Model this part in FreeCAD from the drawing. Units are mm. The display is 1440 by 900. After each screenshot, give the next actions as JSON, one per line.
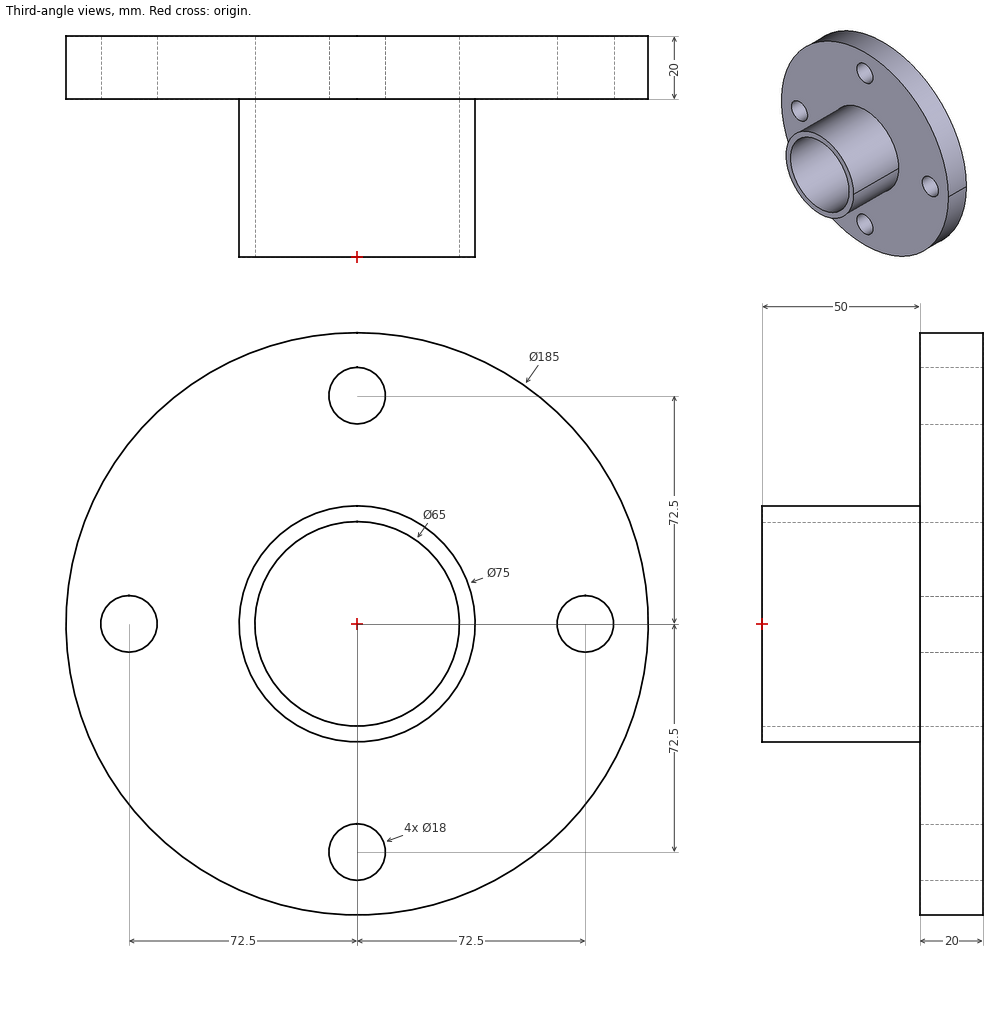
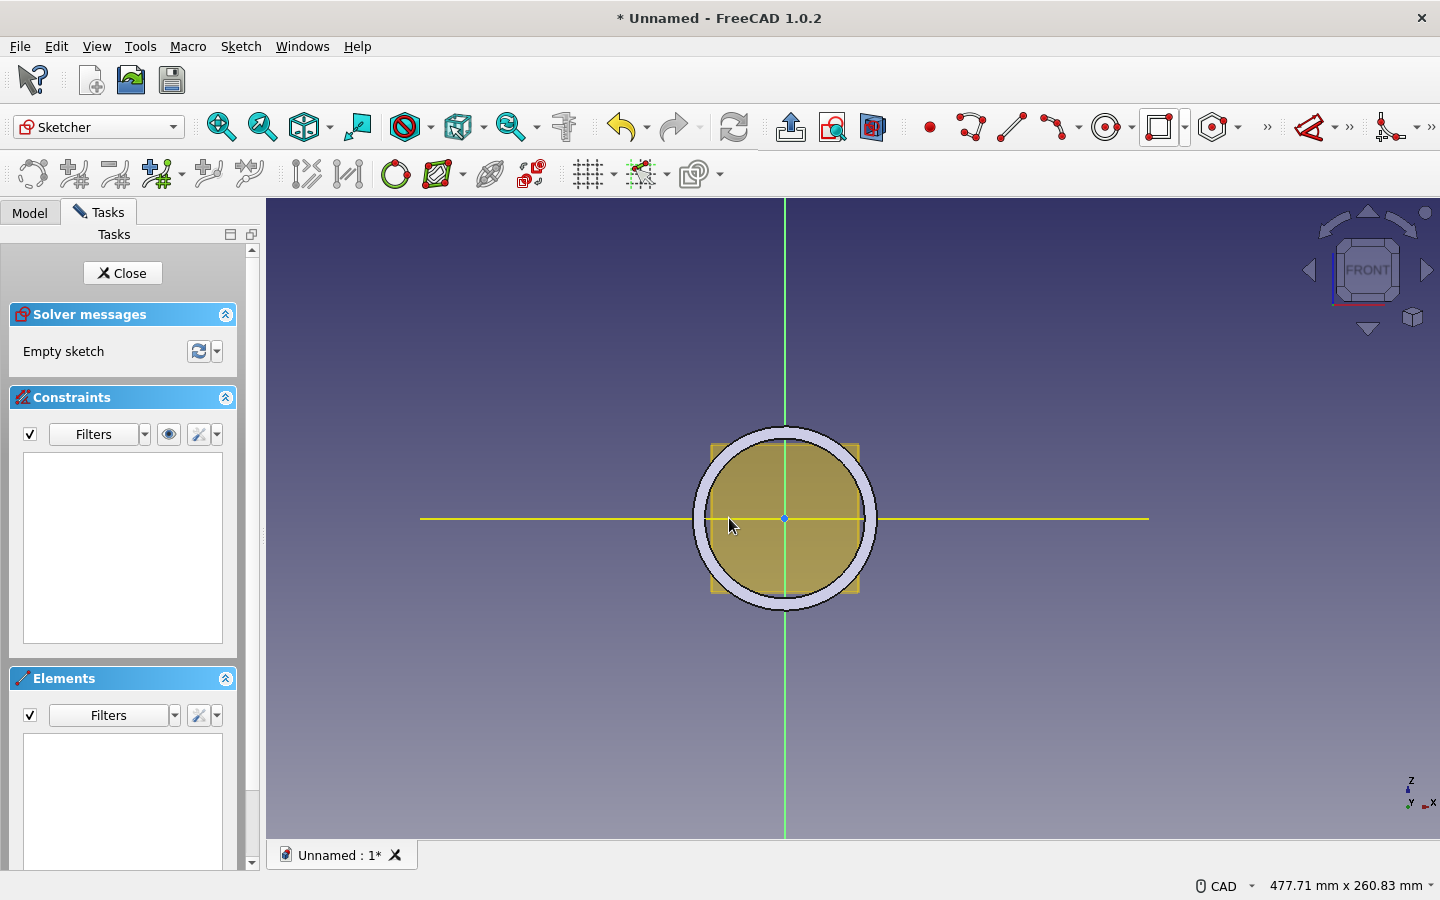
{"action": "left_click", "coordinate": [1106, 128]}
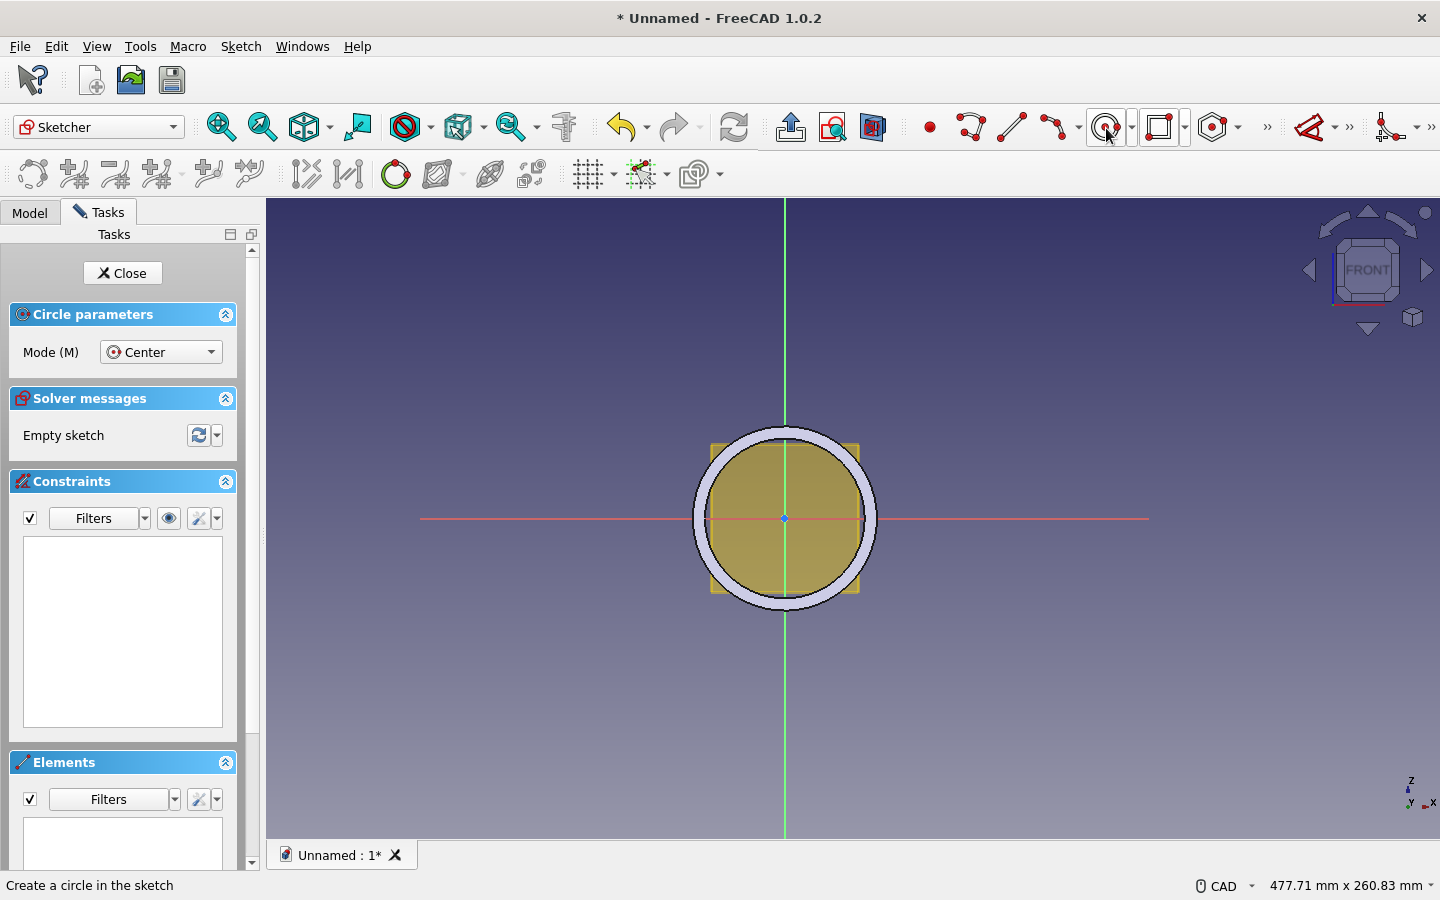
{"action": "left_click", "coordinate": [785, 519]}
{"action": "left_click", "coordinate": [946, 358]}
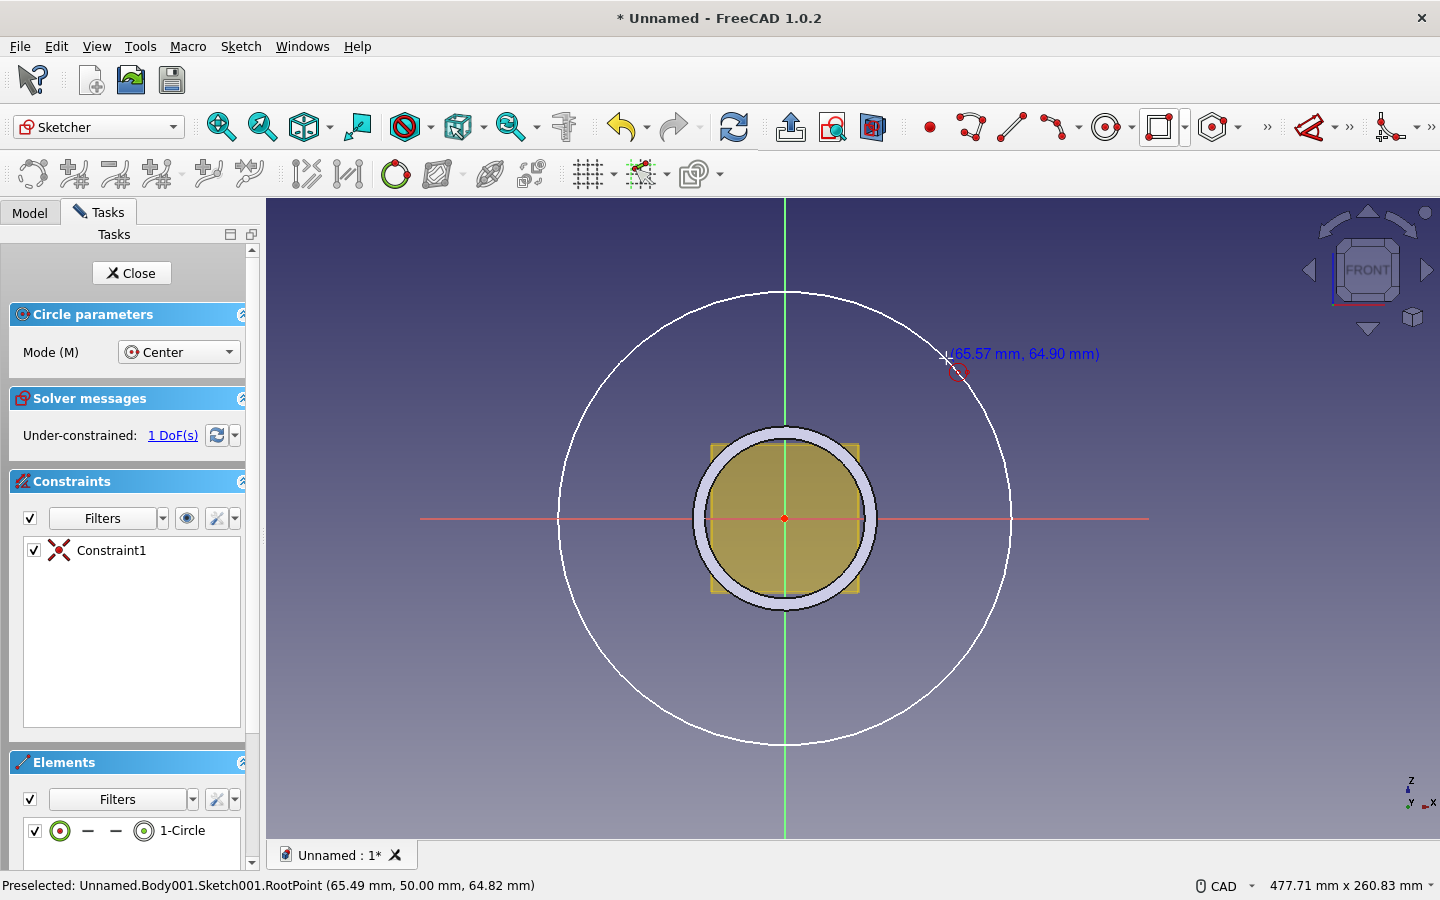
{"action": "left_click", "coordinate": [785, 697]}
{"action": "left_click", "coordinate": [800, 681]}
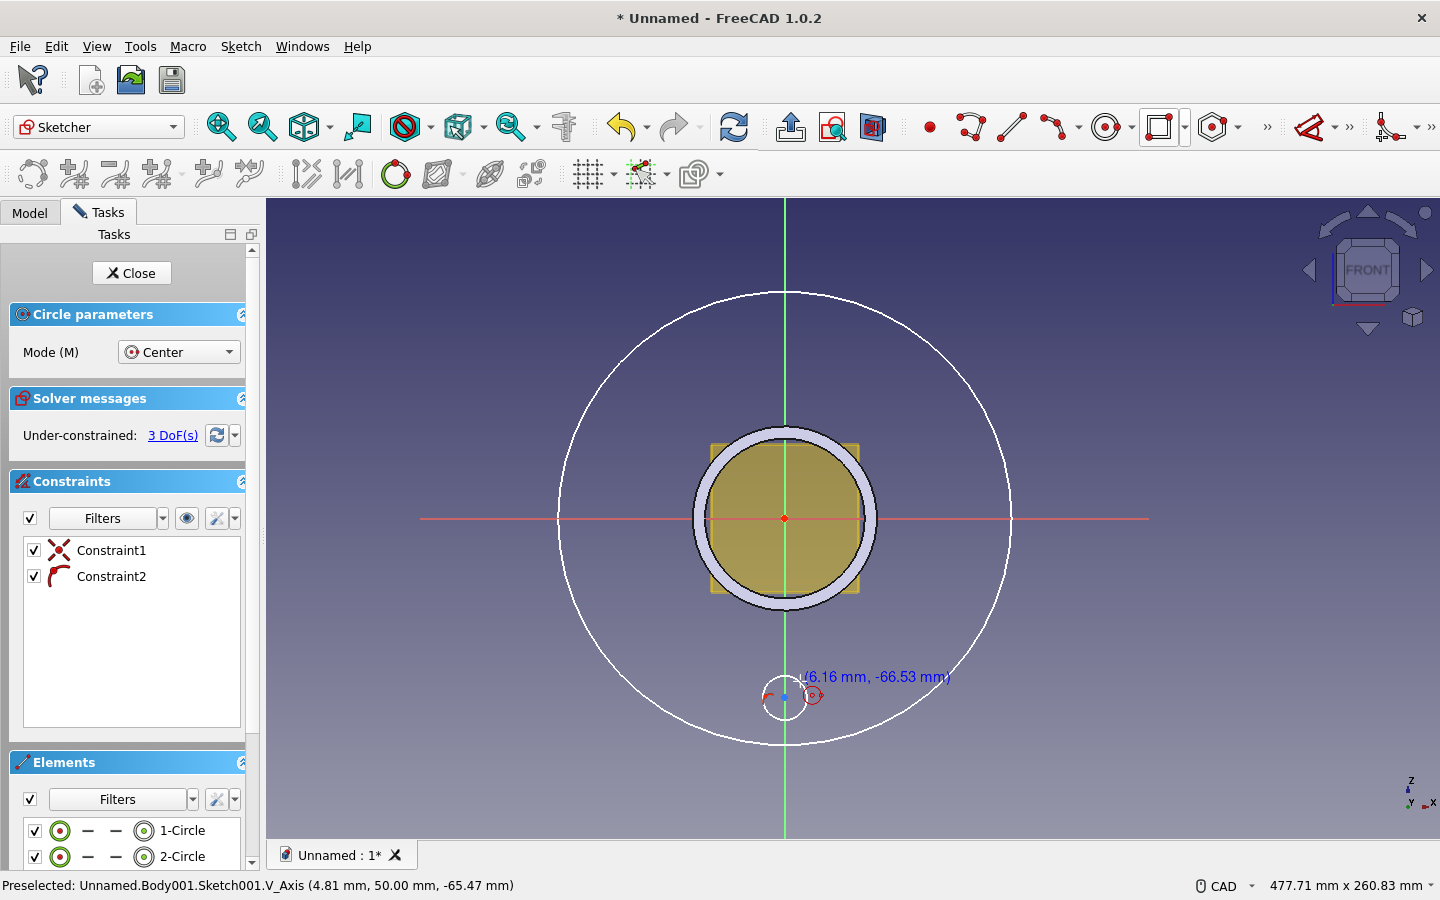
{"action": "left_click", "coordinate": [607, 519]}
{"action": "left_click", "coordinate": [622, 503]}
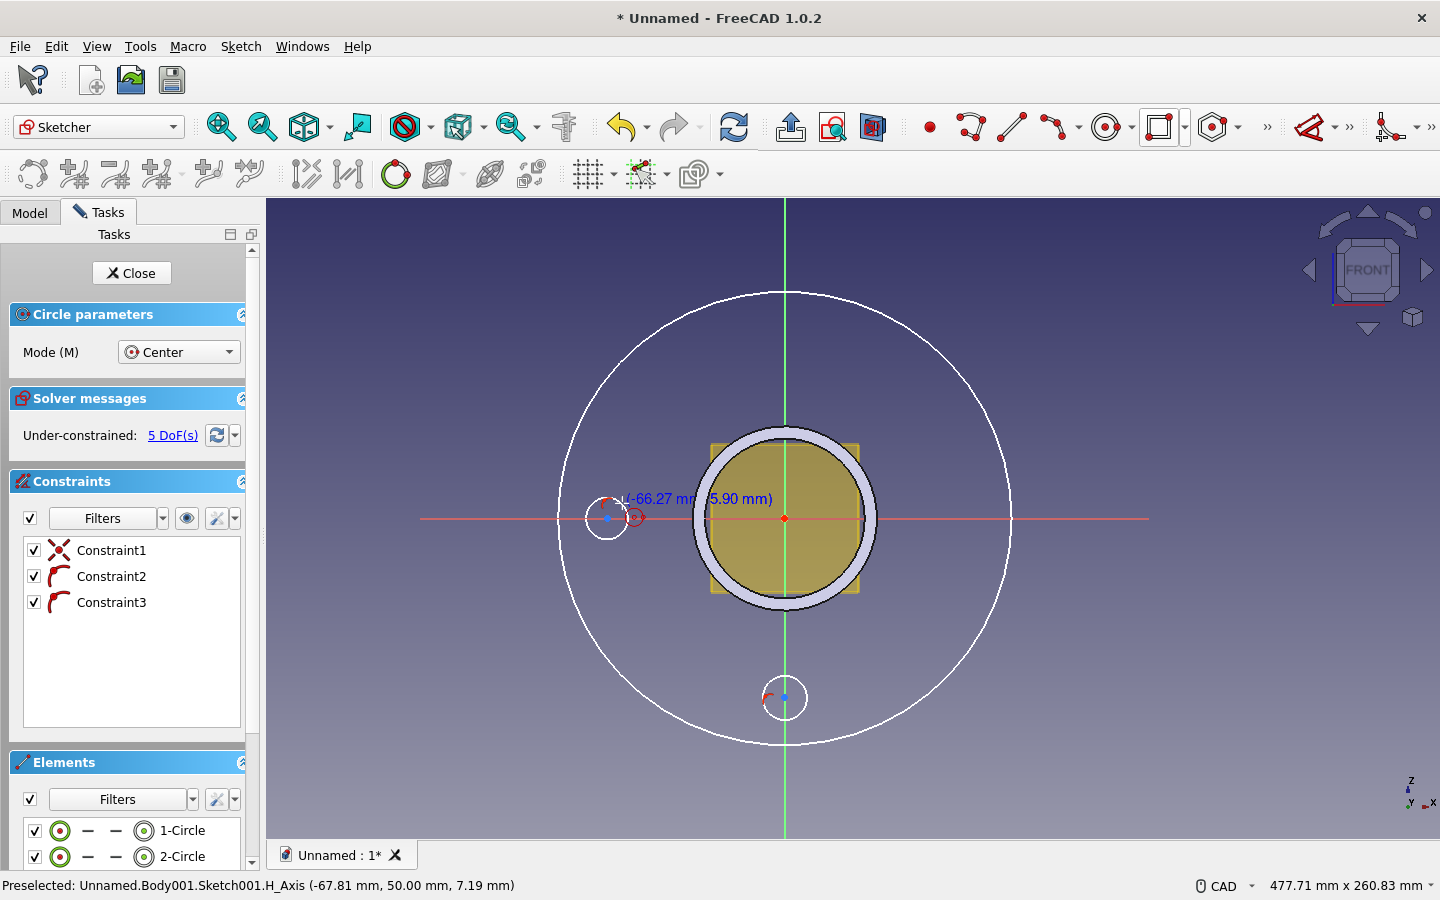
{"action": "left_click", "coordinate": [963, 519]}
{"action": "left_click", "coordinate": [979, 503]}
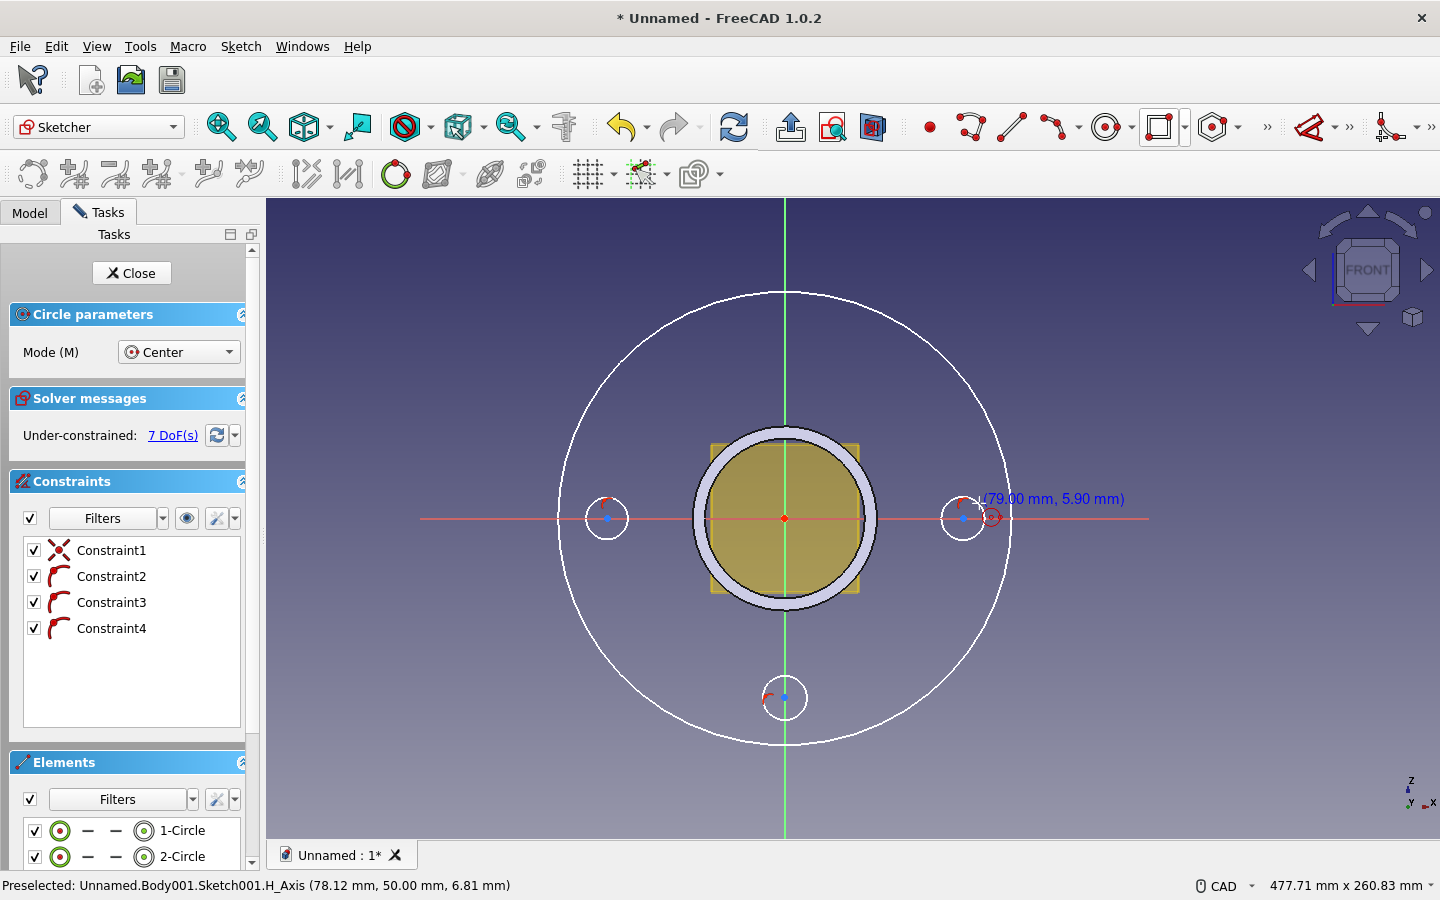
{"action": "left_click", "coordinate": [785, 519]}
{"action": "left_click", "coordinate": [850, 453]}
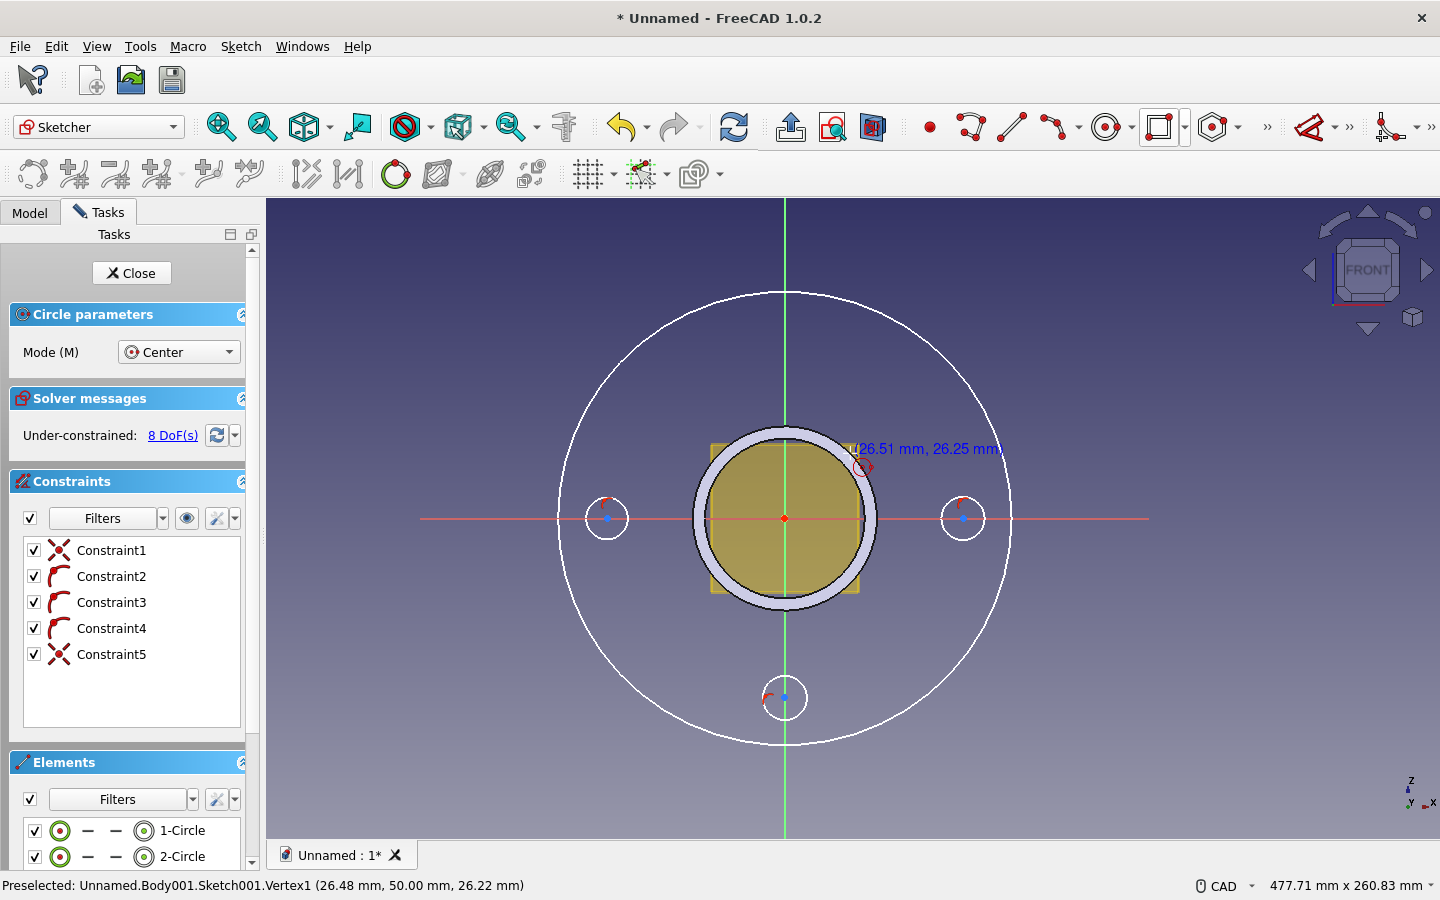
{"action": "left_click", "coordinate": [785, 340]}
{"action": "left_click", "coordinate": [800, 325]}
{"action": "key", "text": "Escape"}